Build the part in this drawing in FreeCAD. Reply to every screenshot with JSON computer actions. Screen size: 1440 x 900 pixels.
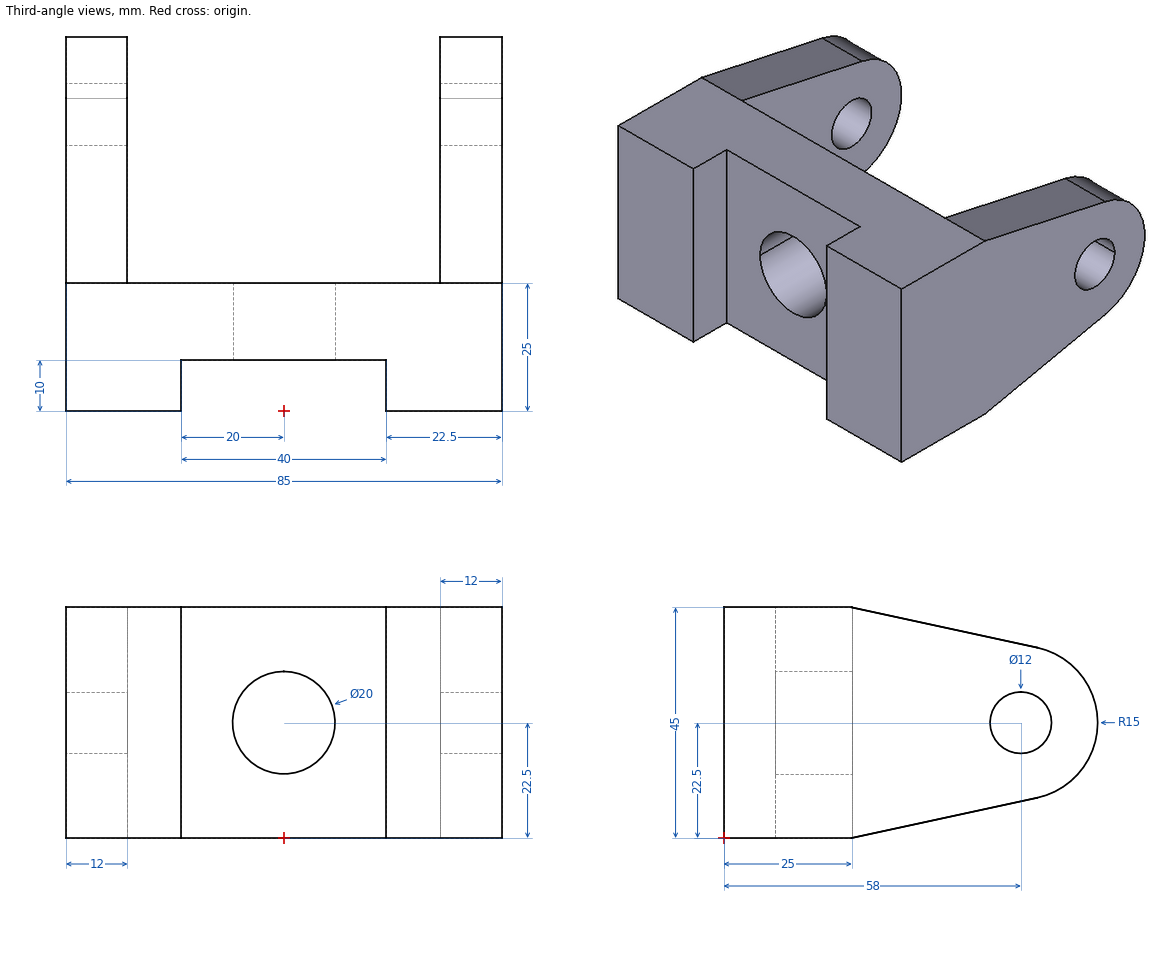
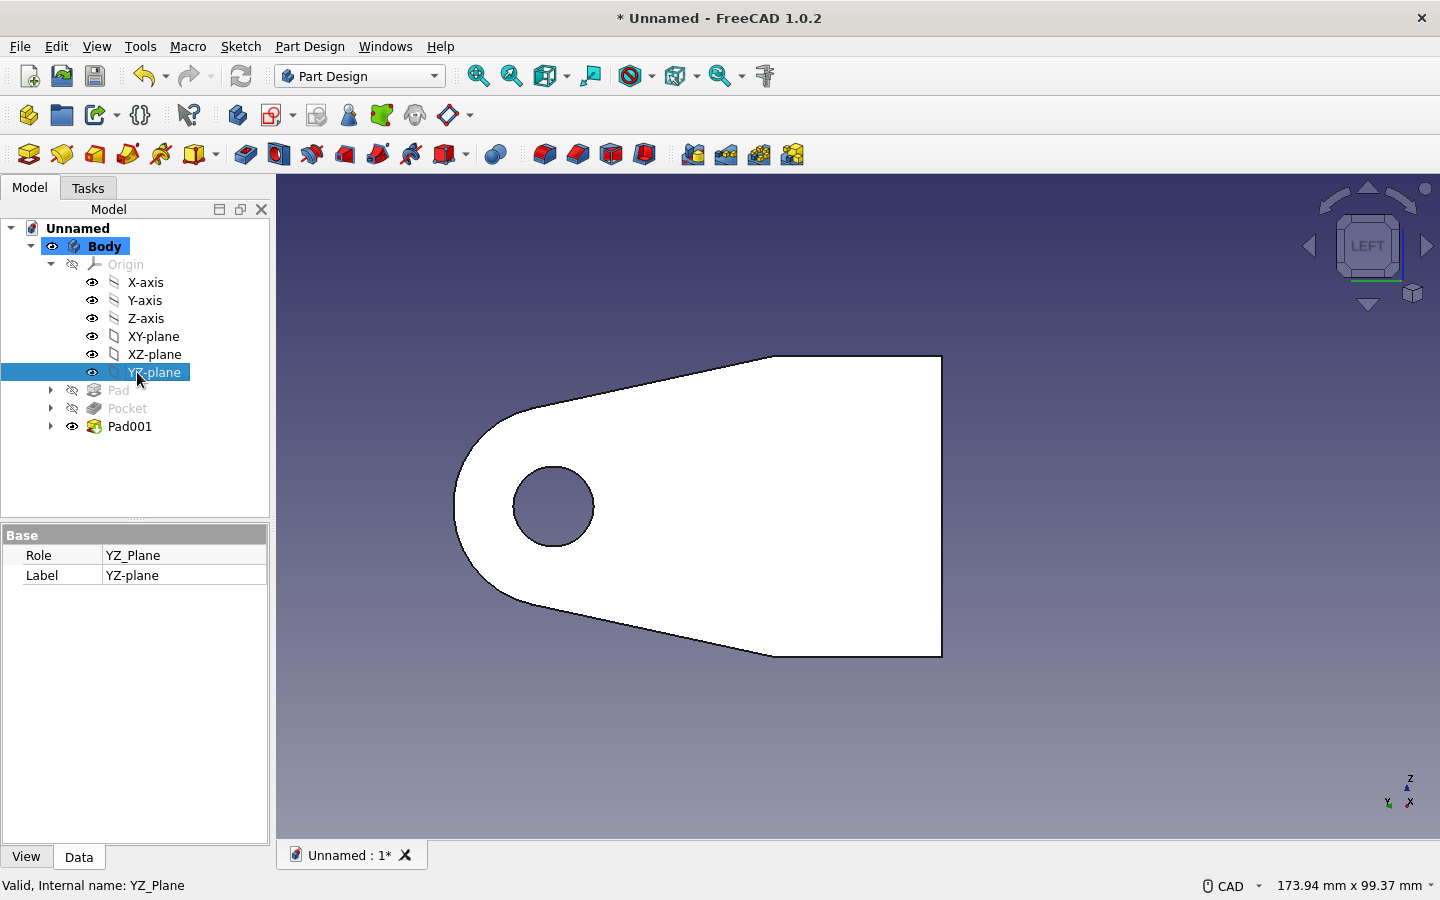
{"action": "left_click", "coordinate": [448, 116]}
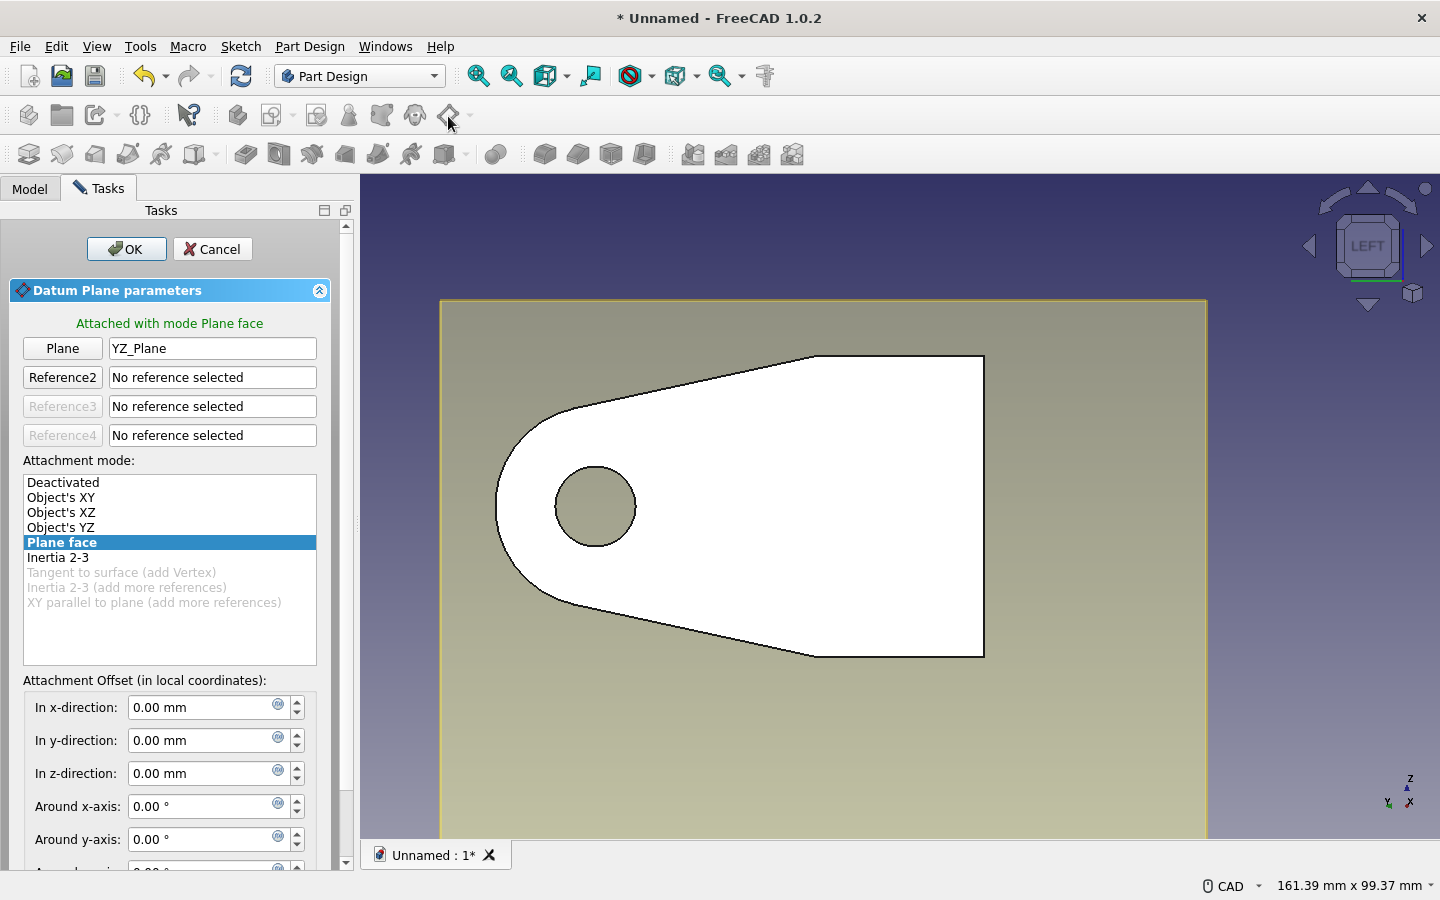
{"action": "triple_click", "coordinate": [210, 774]}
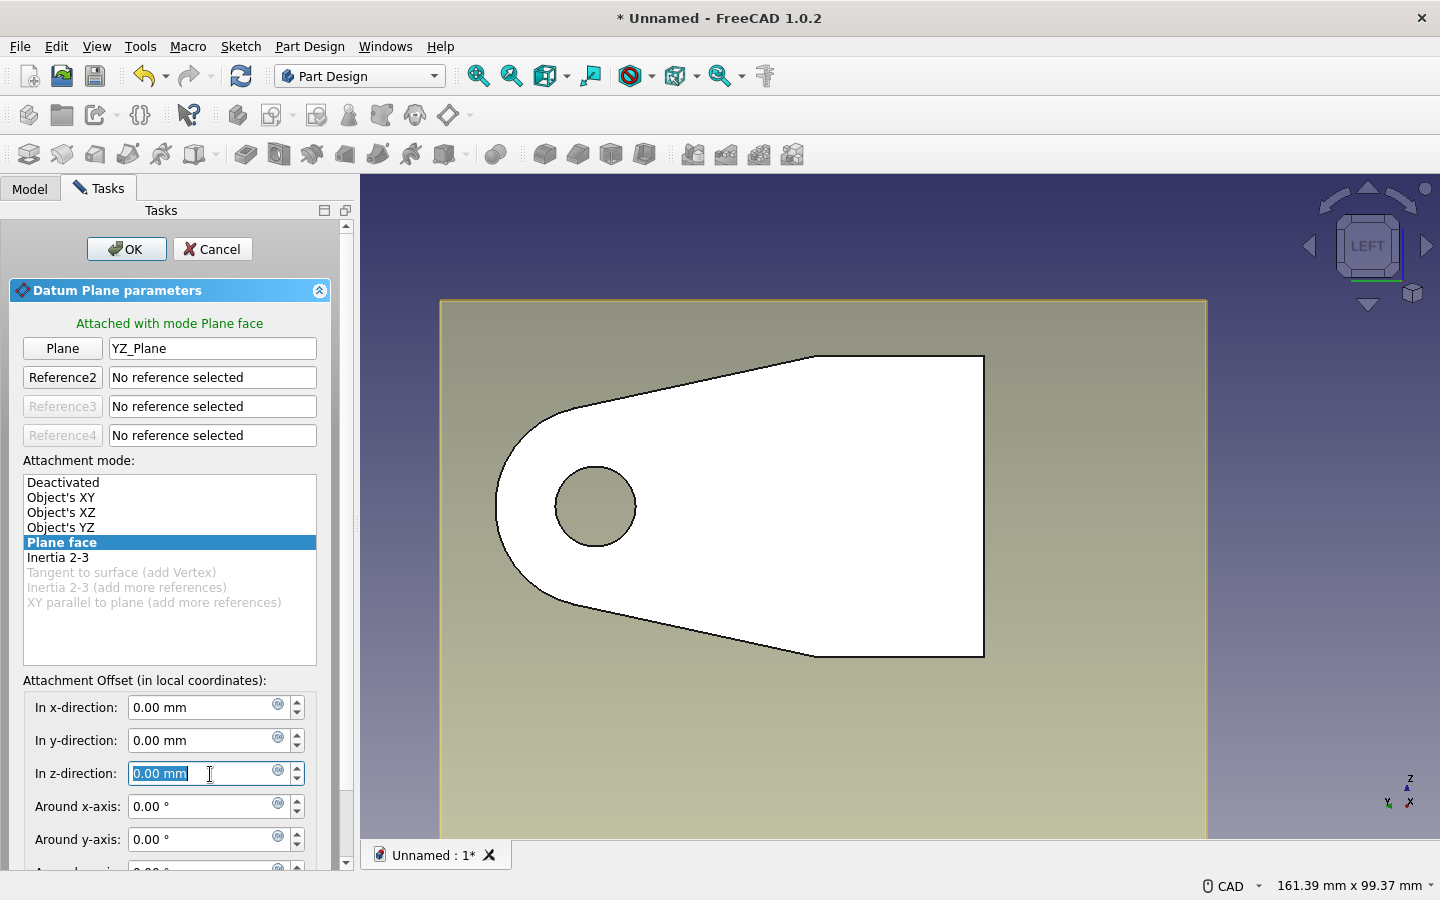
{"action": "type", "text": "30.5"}
{"action": "key", "text": "Tab"}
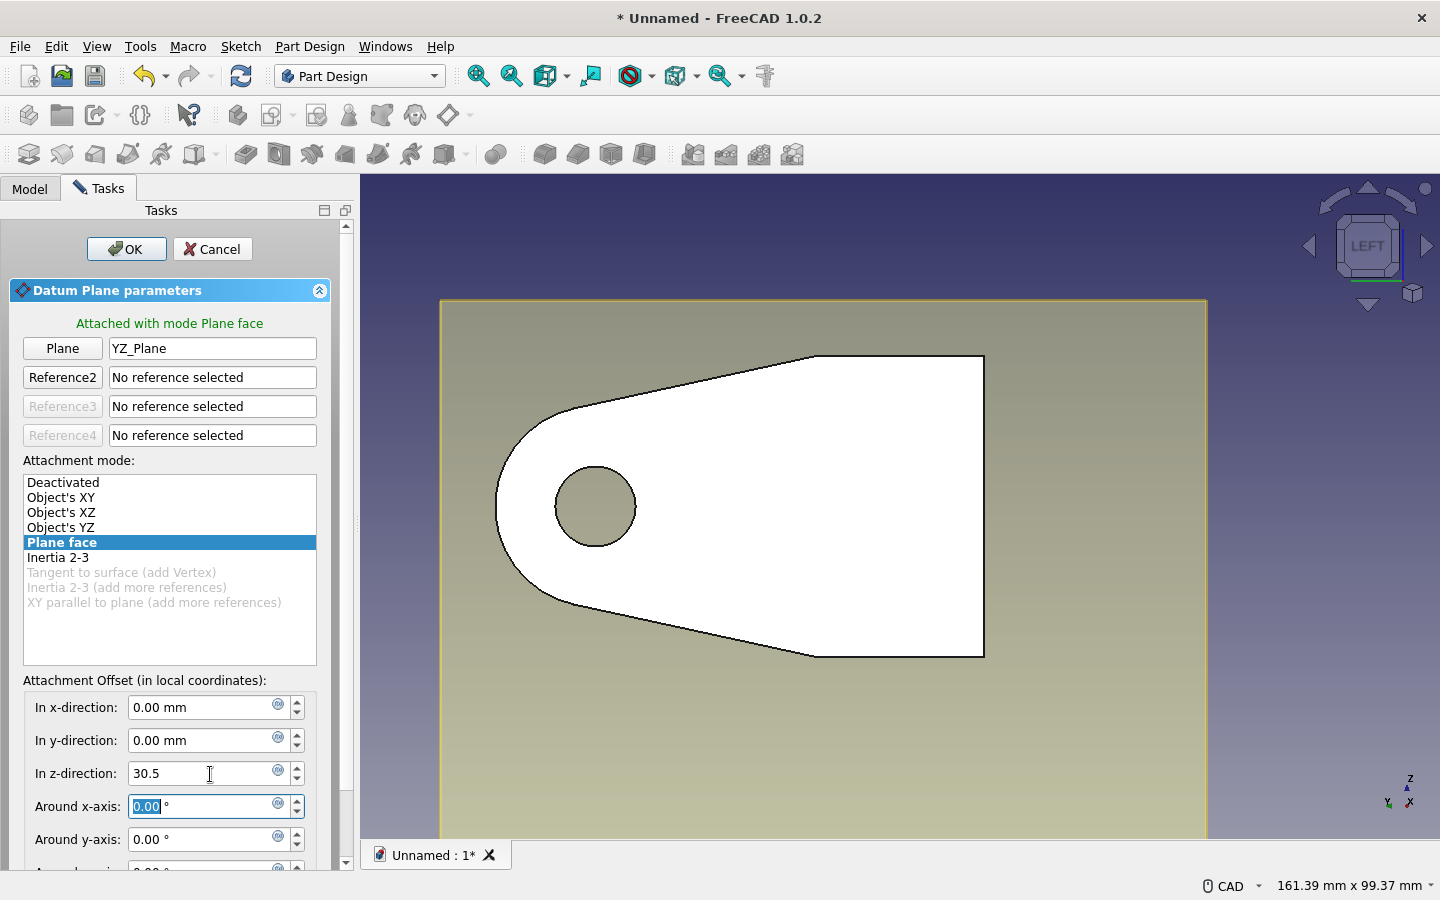
{"action": "left_click", "coordinate": [127, 249]}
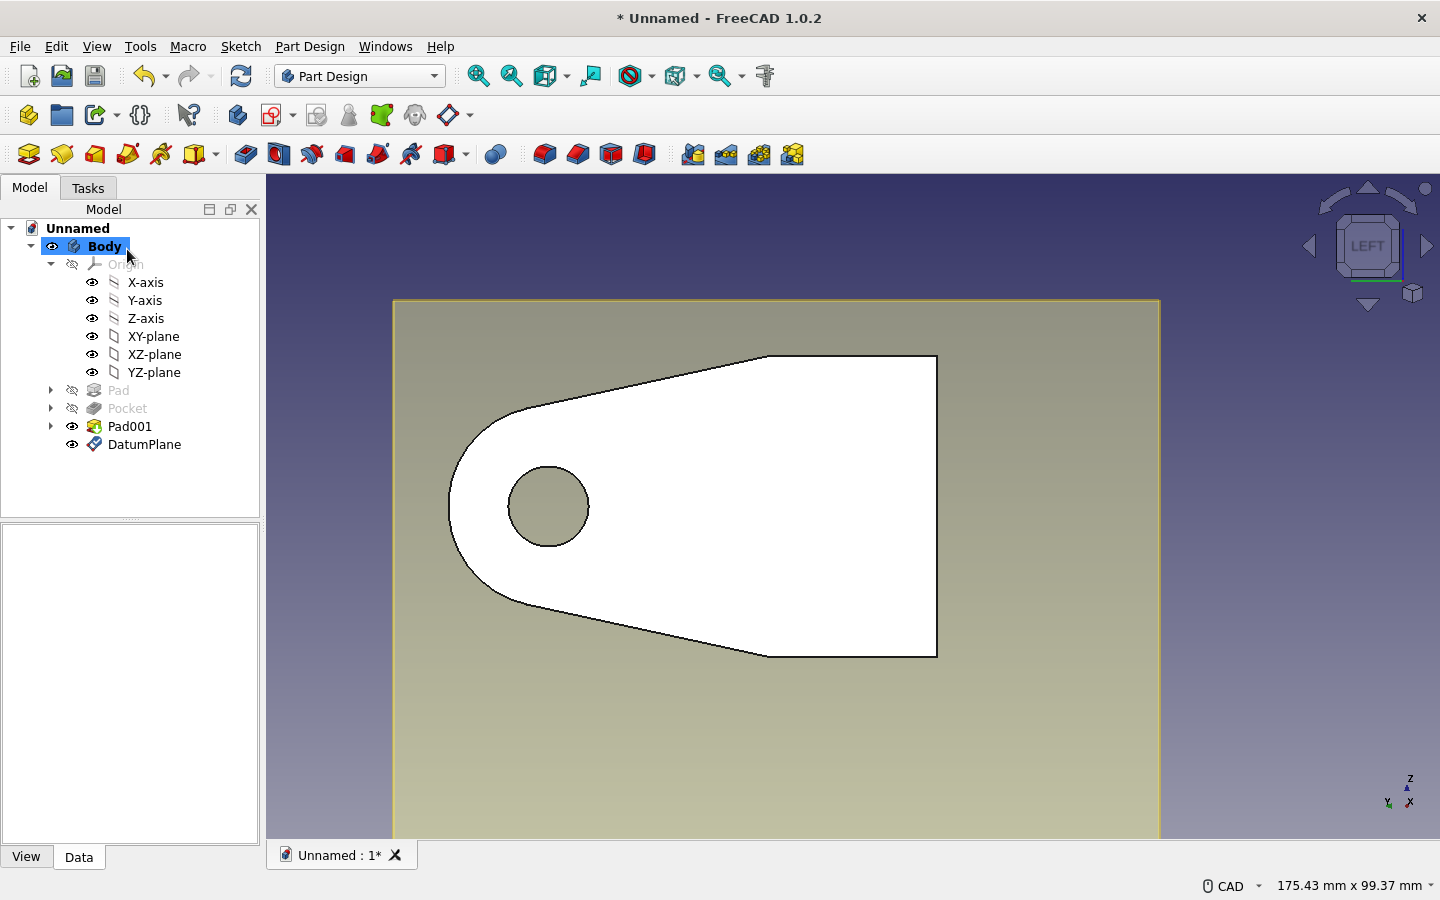
{"action": "left_click", "coordinate": [117, 444]}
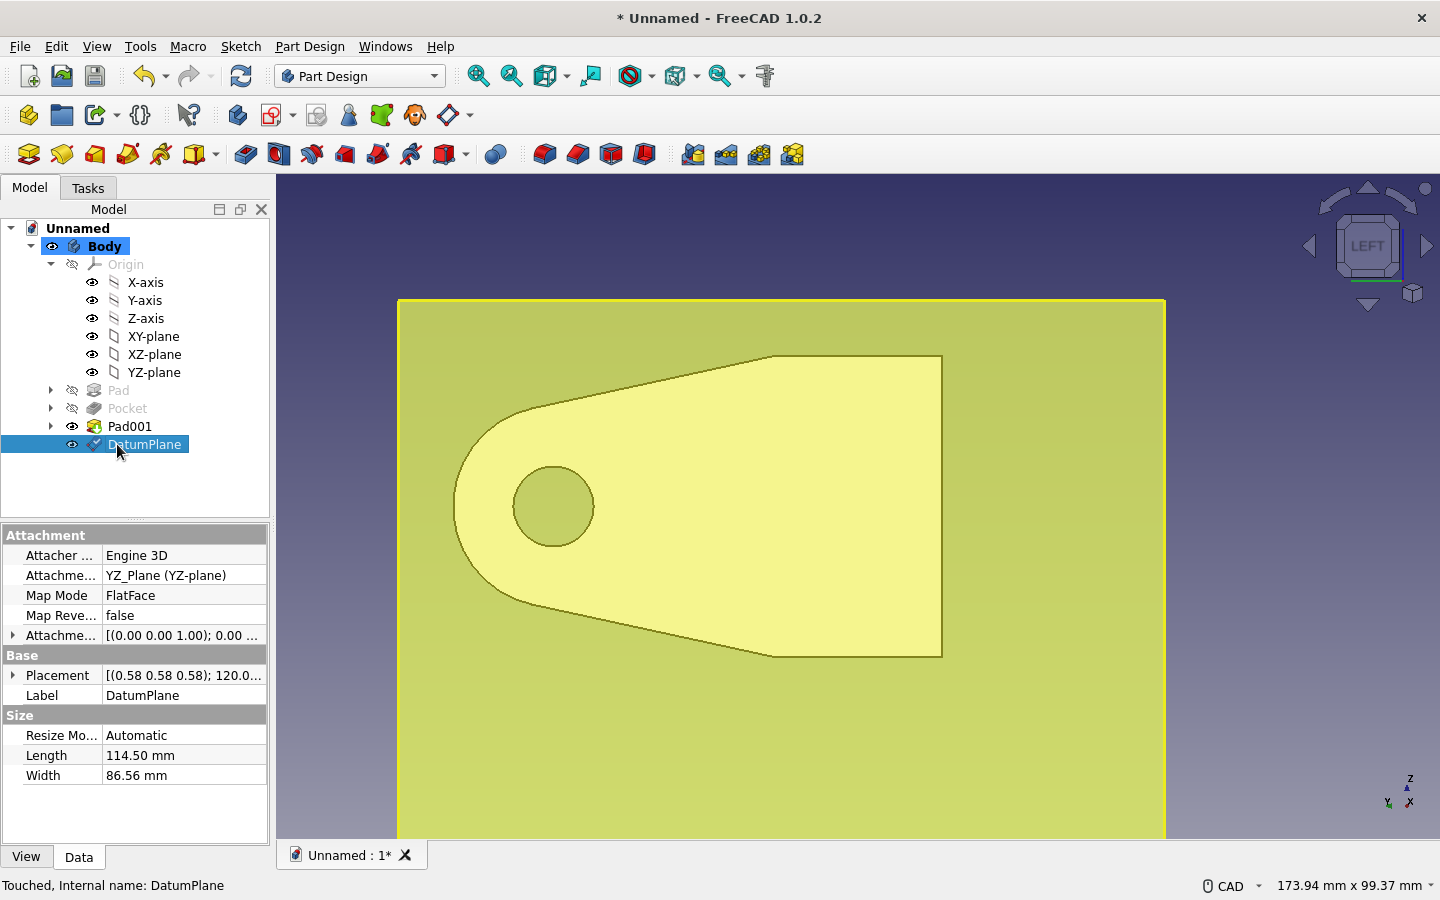
{"action": "left_click", "coordinate": [270, 116]}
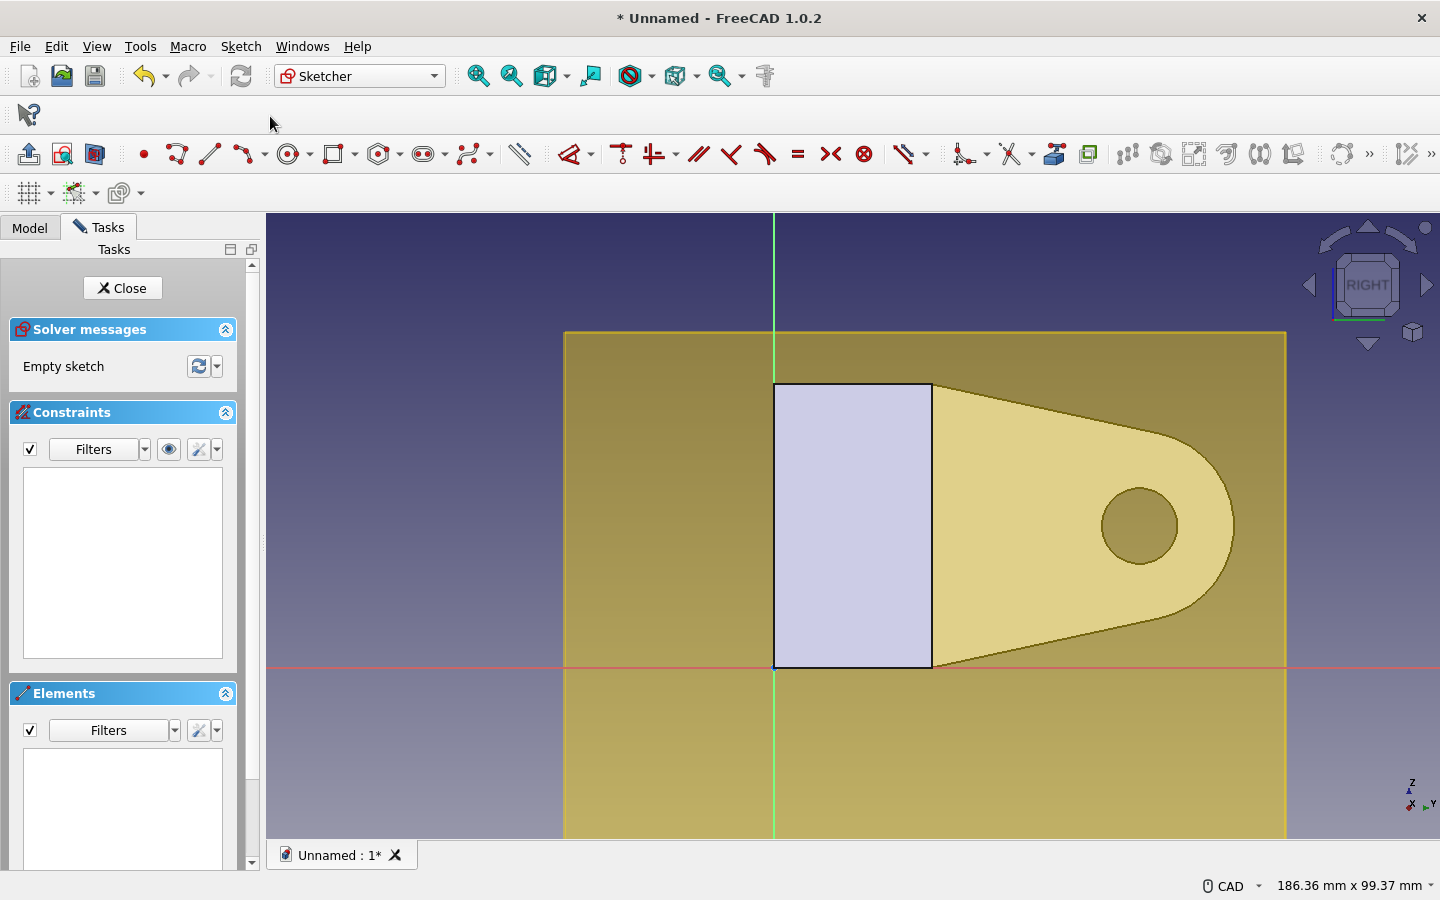
{"action": "left_click", "coordinate": [95, 154]}